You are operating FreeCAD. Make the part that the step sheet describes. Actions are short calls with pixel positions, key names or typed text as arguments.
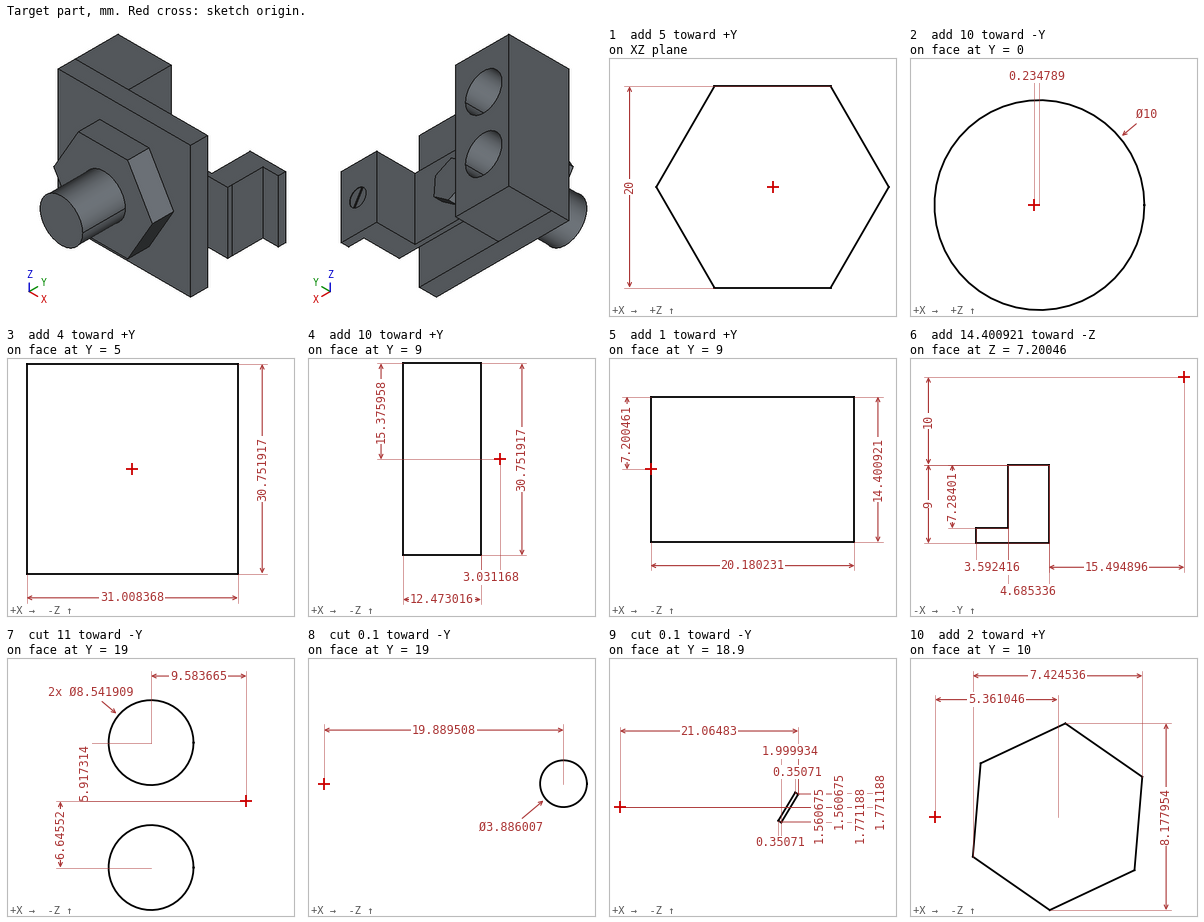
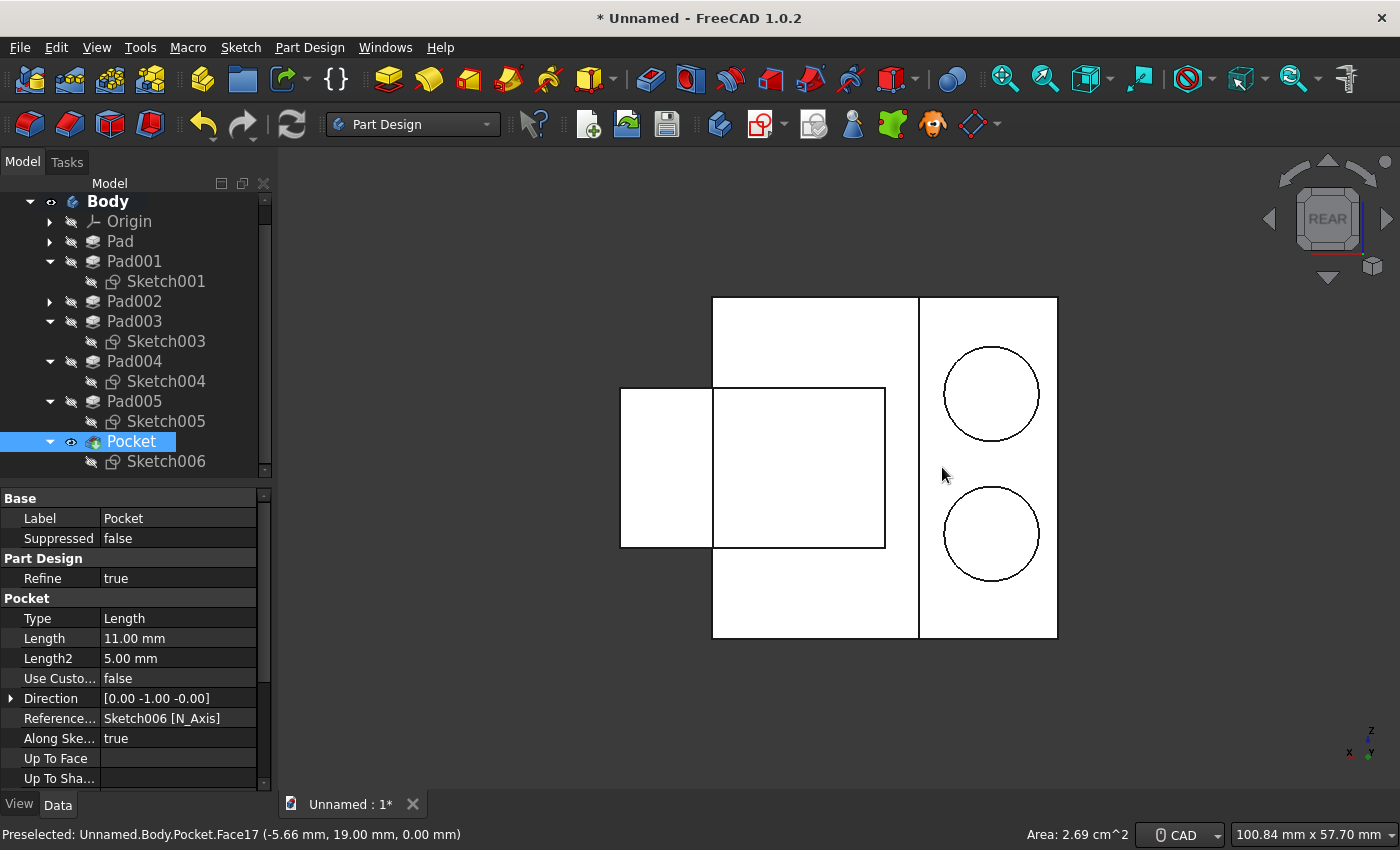
click(760, 124)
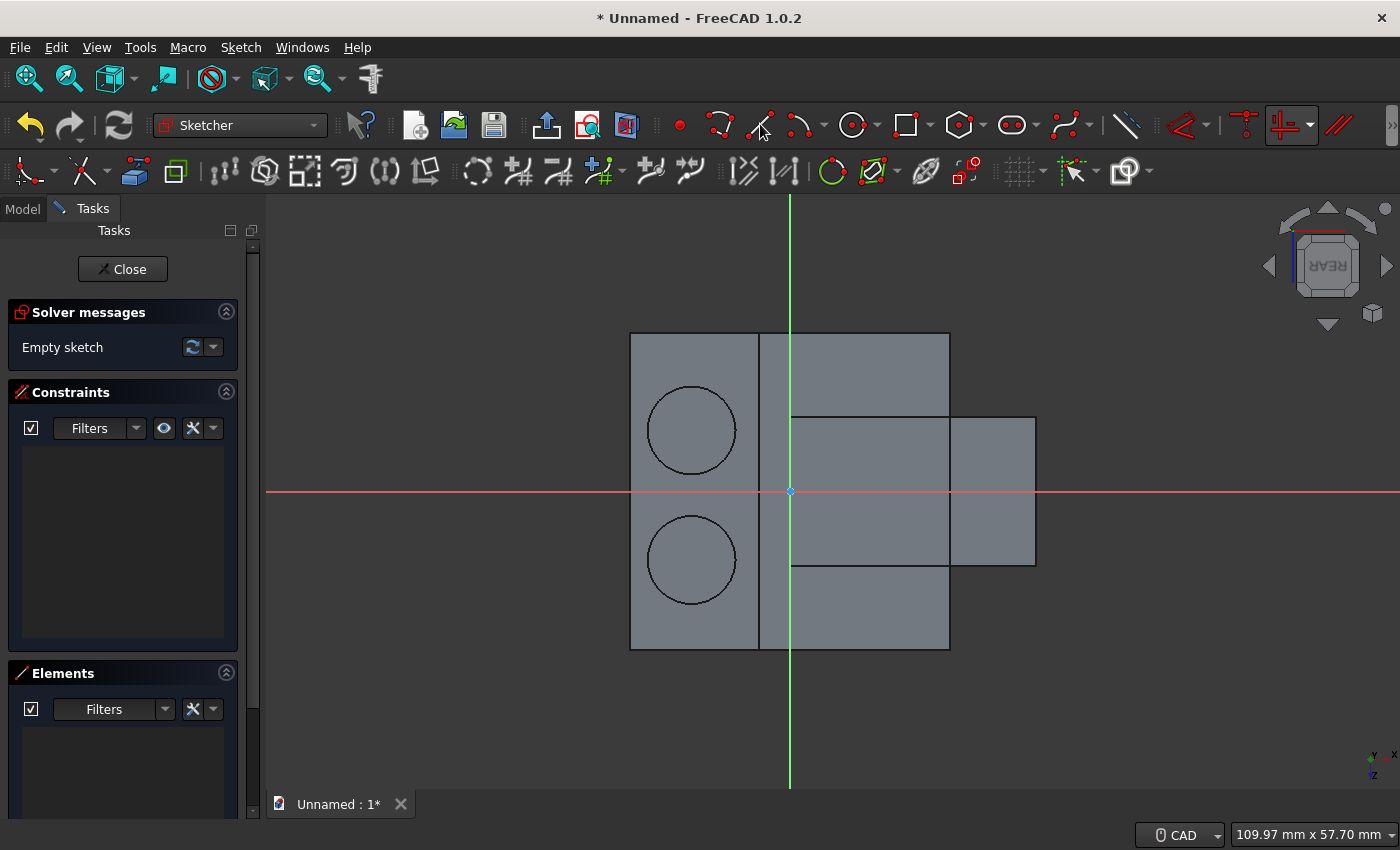
scroll(1024, 491, up, 11)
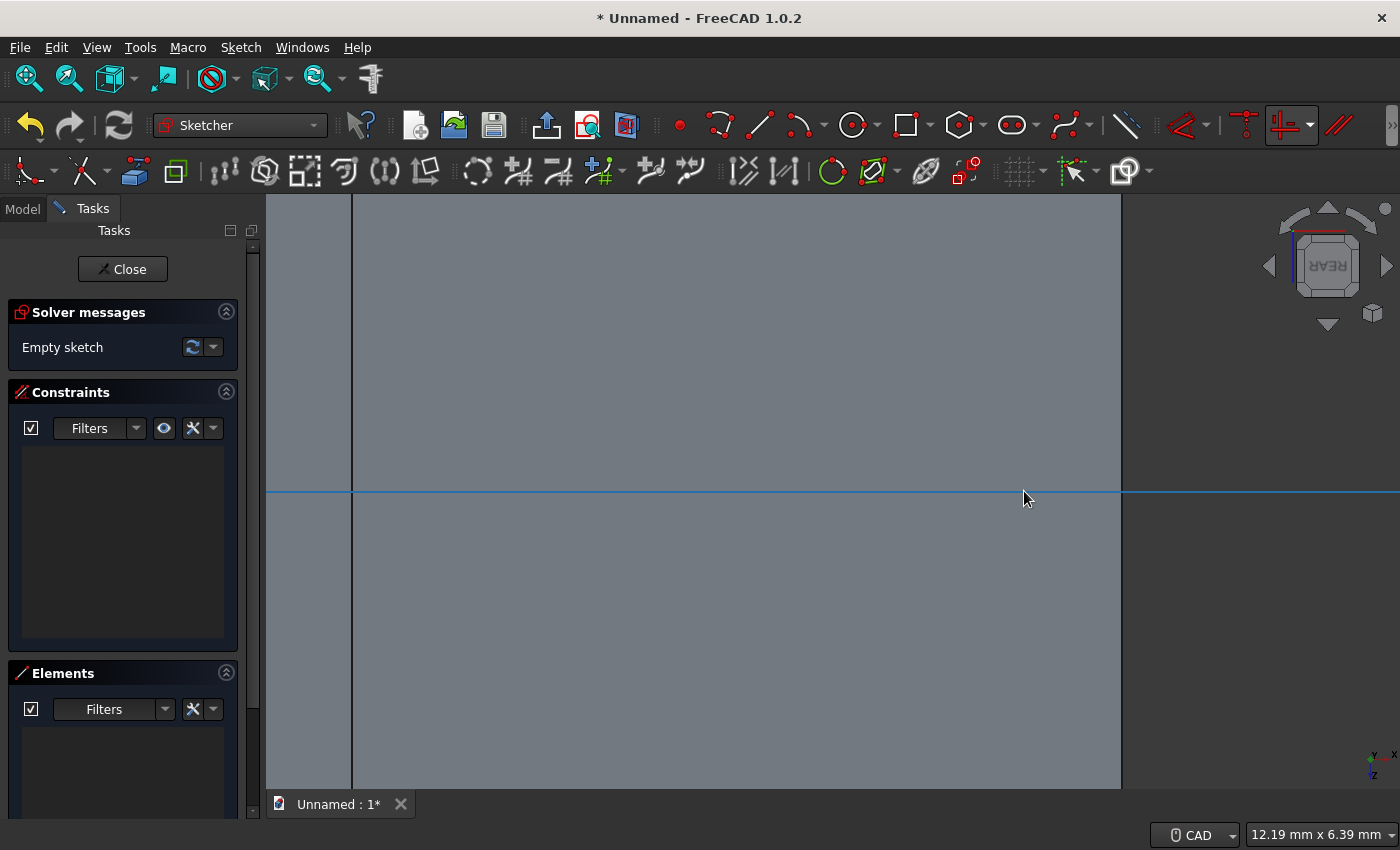
click(854, 126)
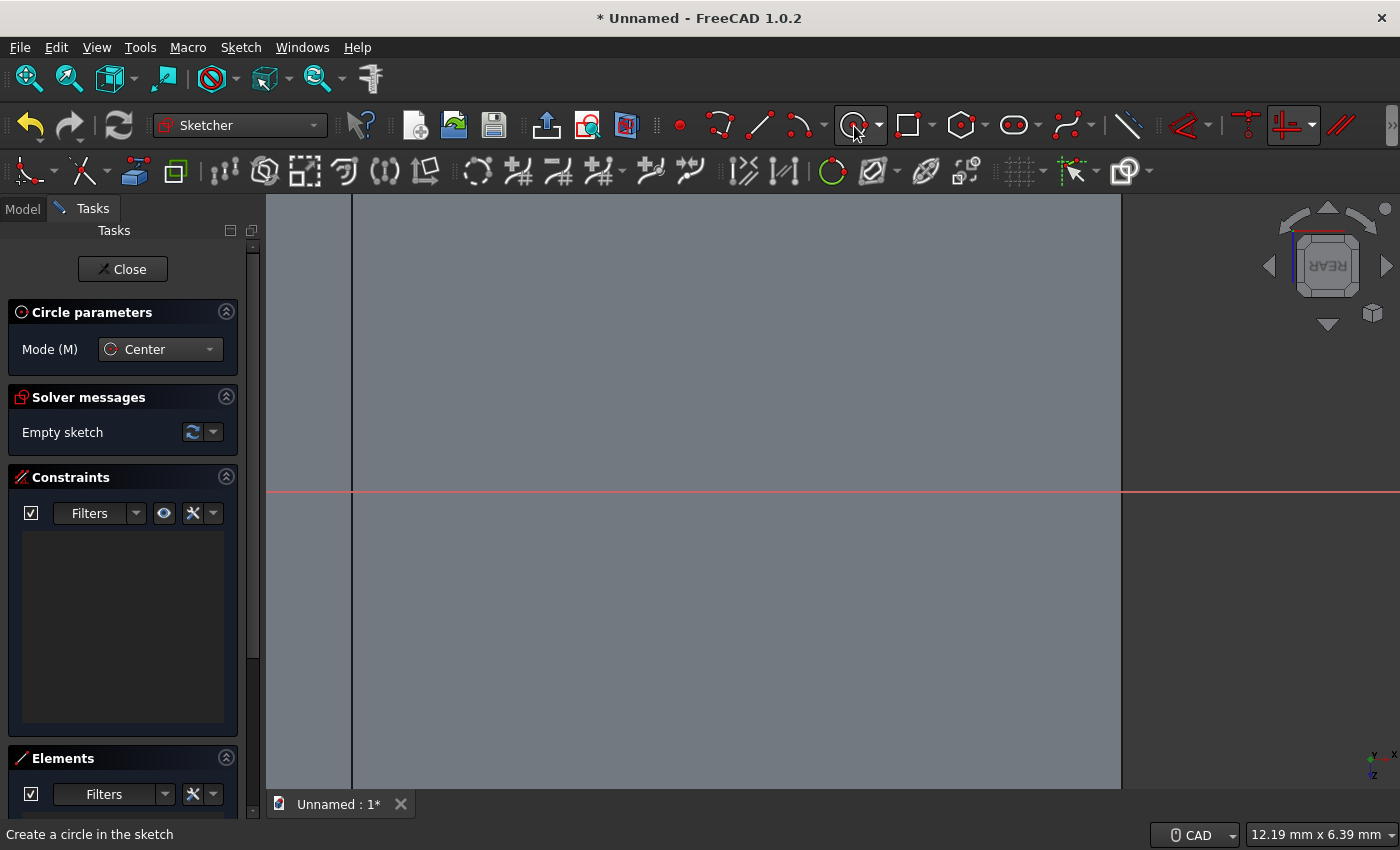
click(761, 491)
move(889, 364)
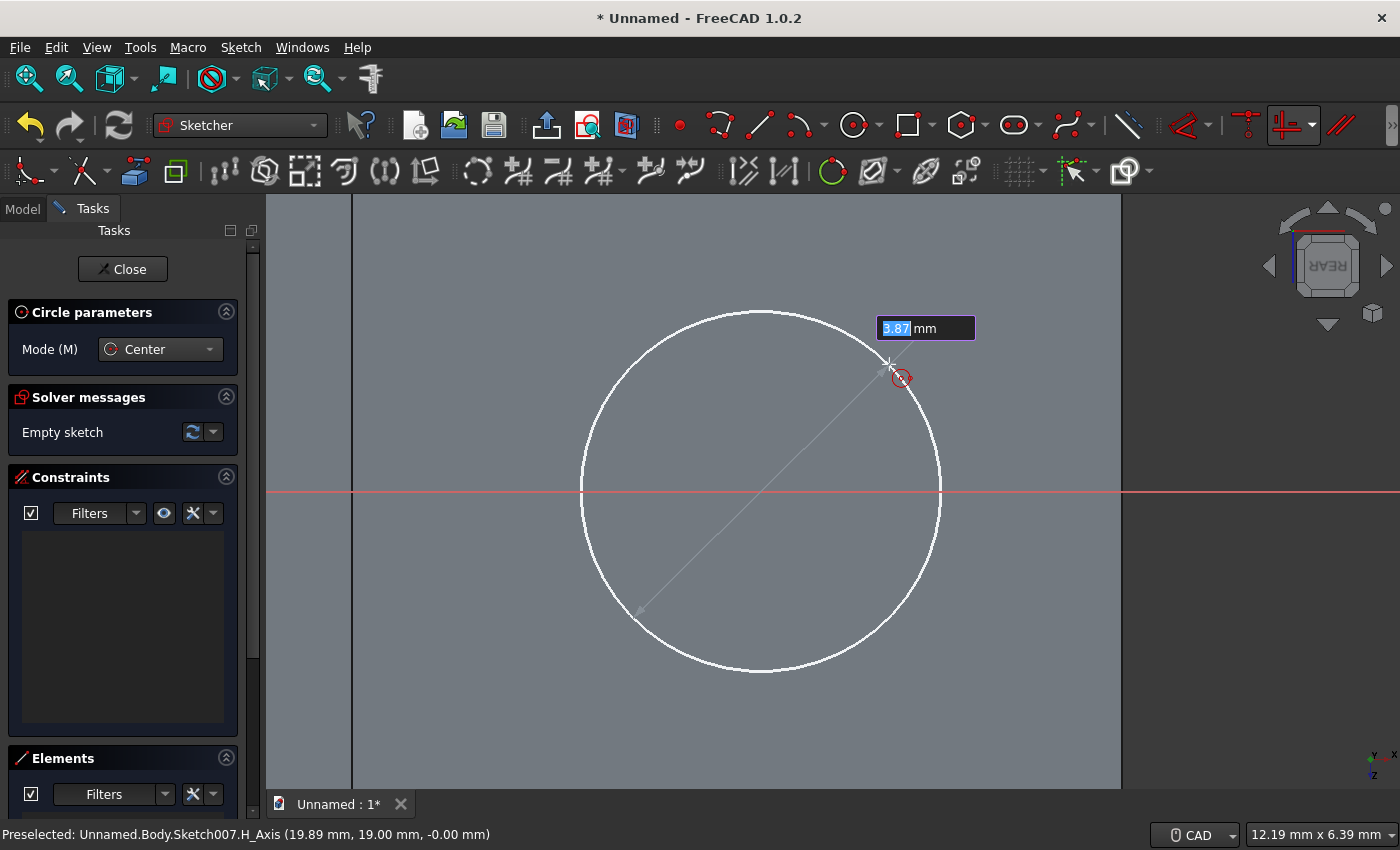
text(3.886007)
key(Return)
key(Escape)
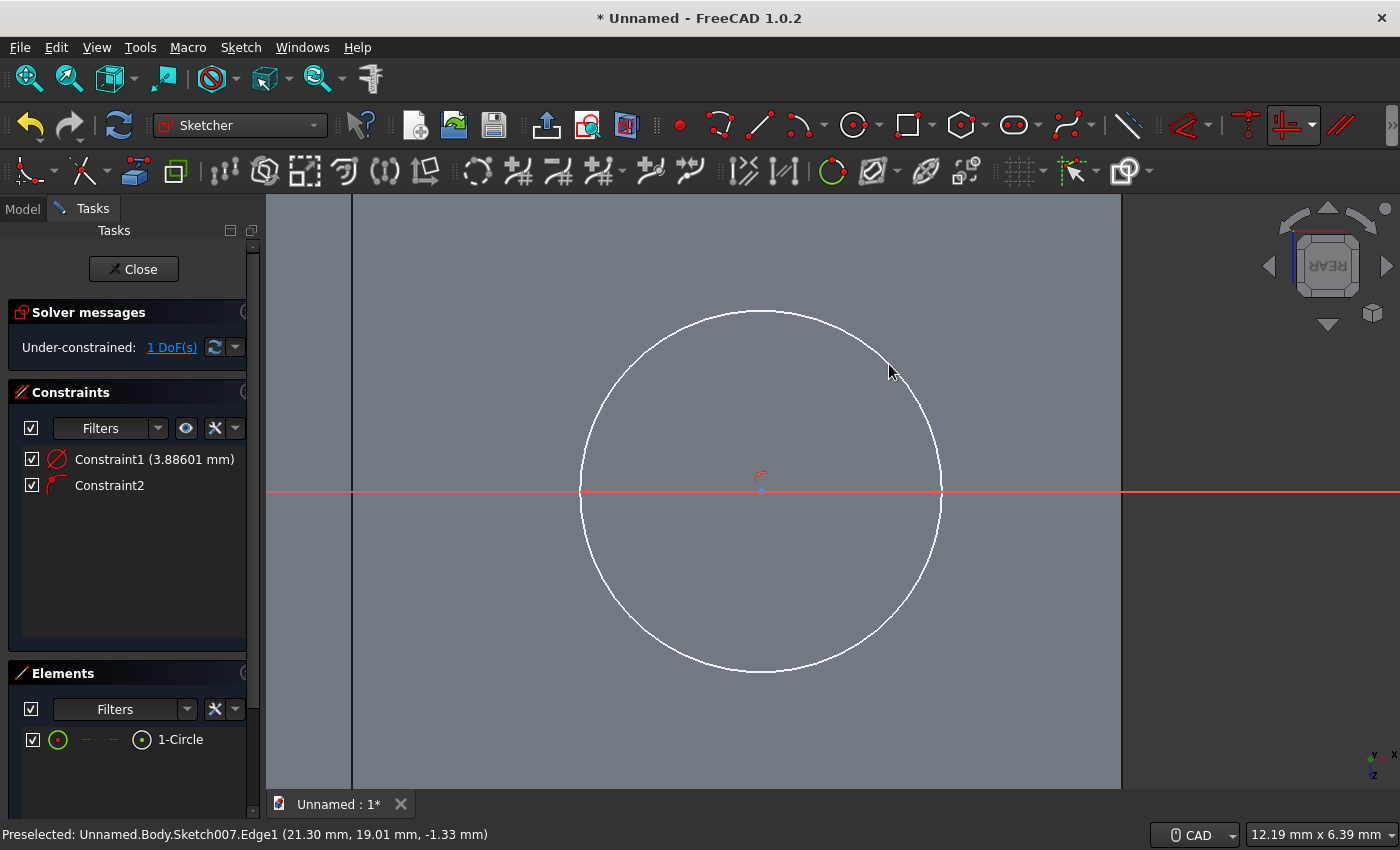
click(1184, 126)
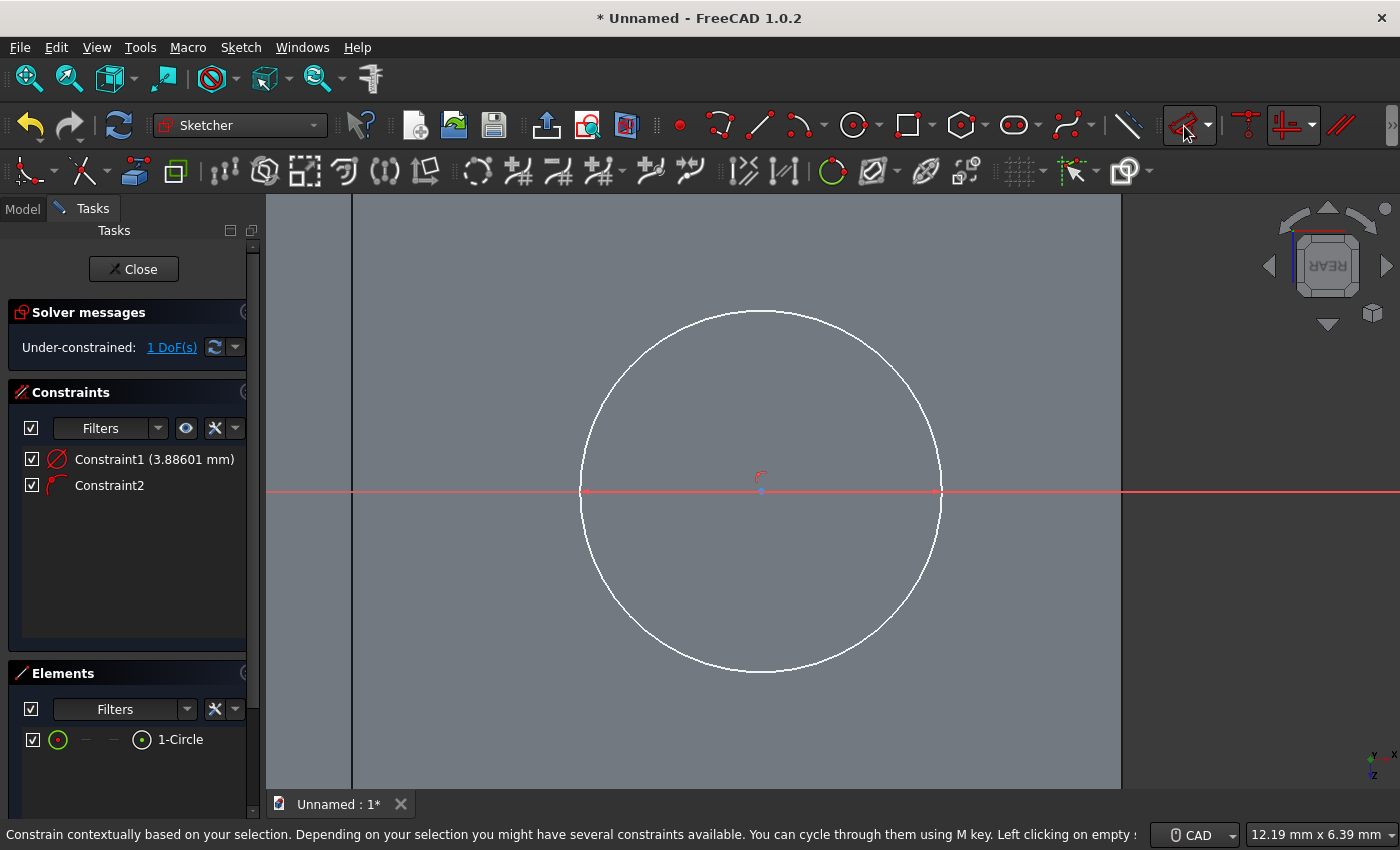
click(761, 491)
click(528, 525)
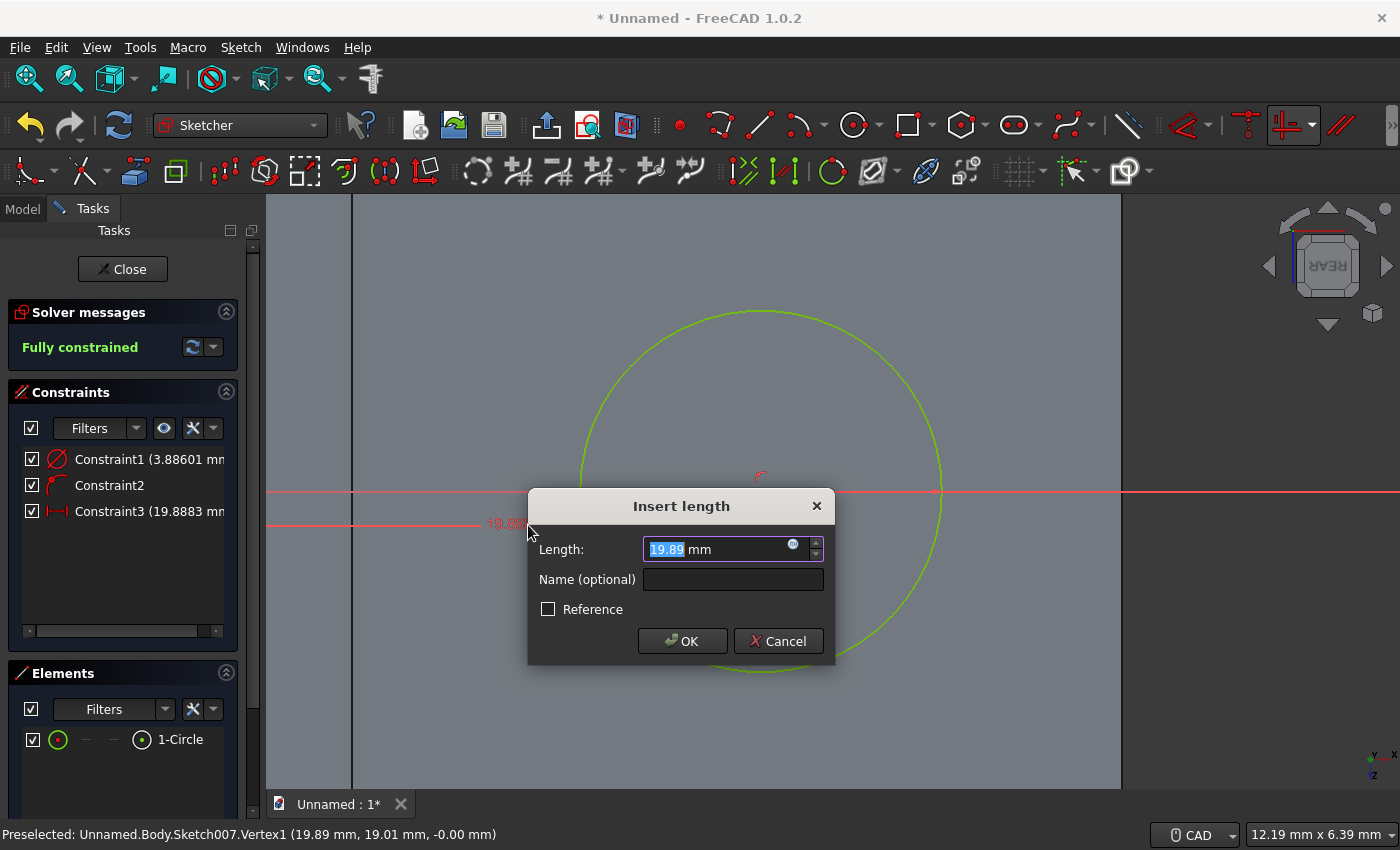
text(19.889508)
key(Return)
key(Escape)